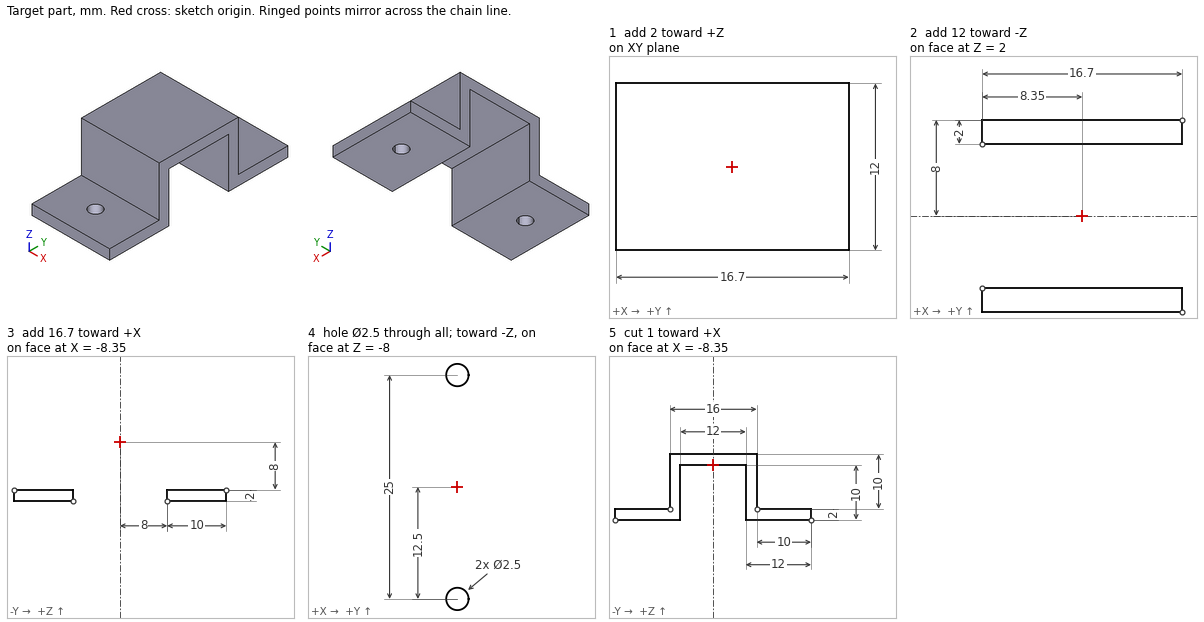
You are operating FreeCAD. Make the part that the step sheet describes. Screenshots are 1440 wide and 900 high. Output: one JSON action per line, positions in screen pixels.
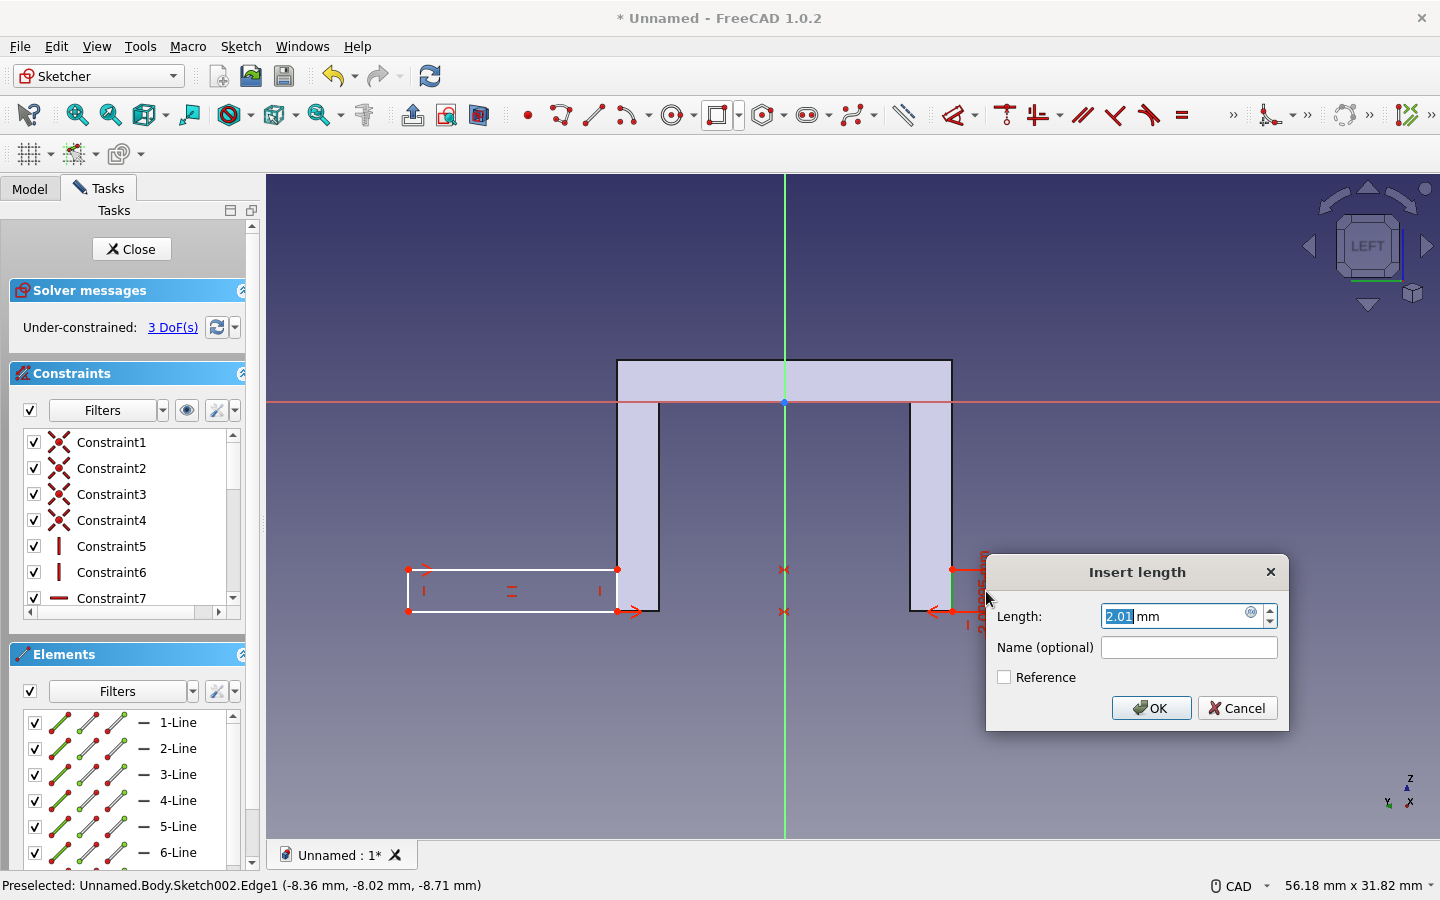
{"action": "type", "text": "2"}
{"action": "key", "text": "Return"}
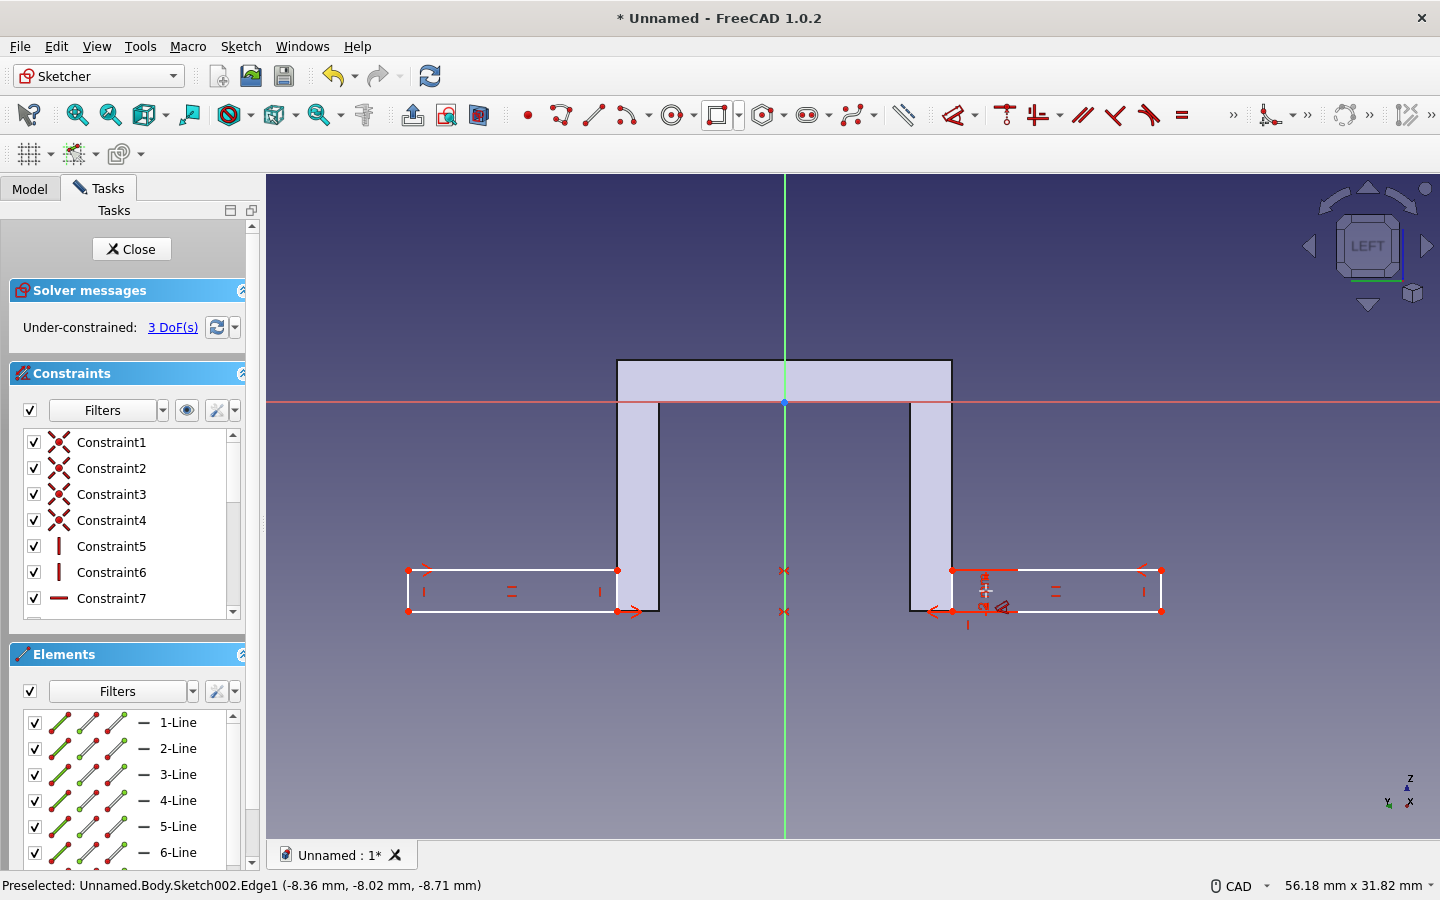
{"action": "left_click", "coordinate": [1015, 612]}
{"action": "left_click", "coordinate": [1057, 646]}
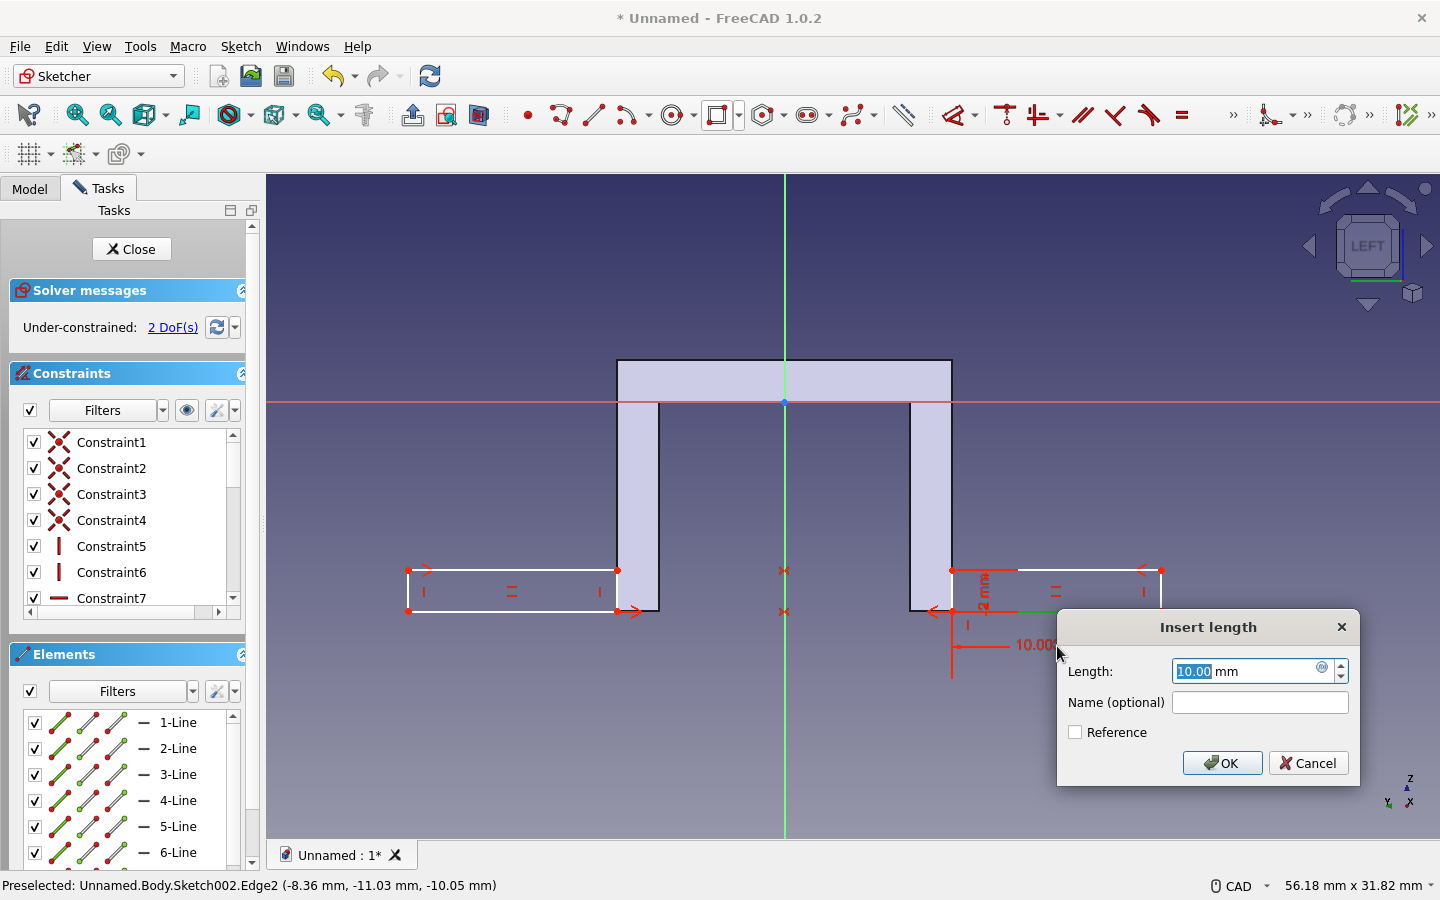
{"action": "type", "text": "10"}
{"action": "key", "text": "Return"}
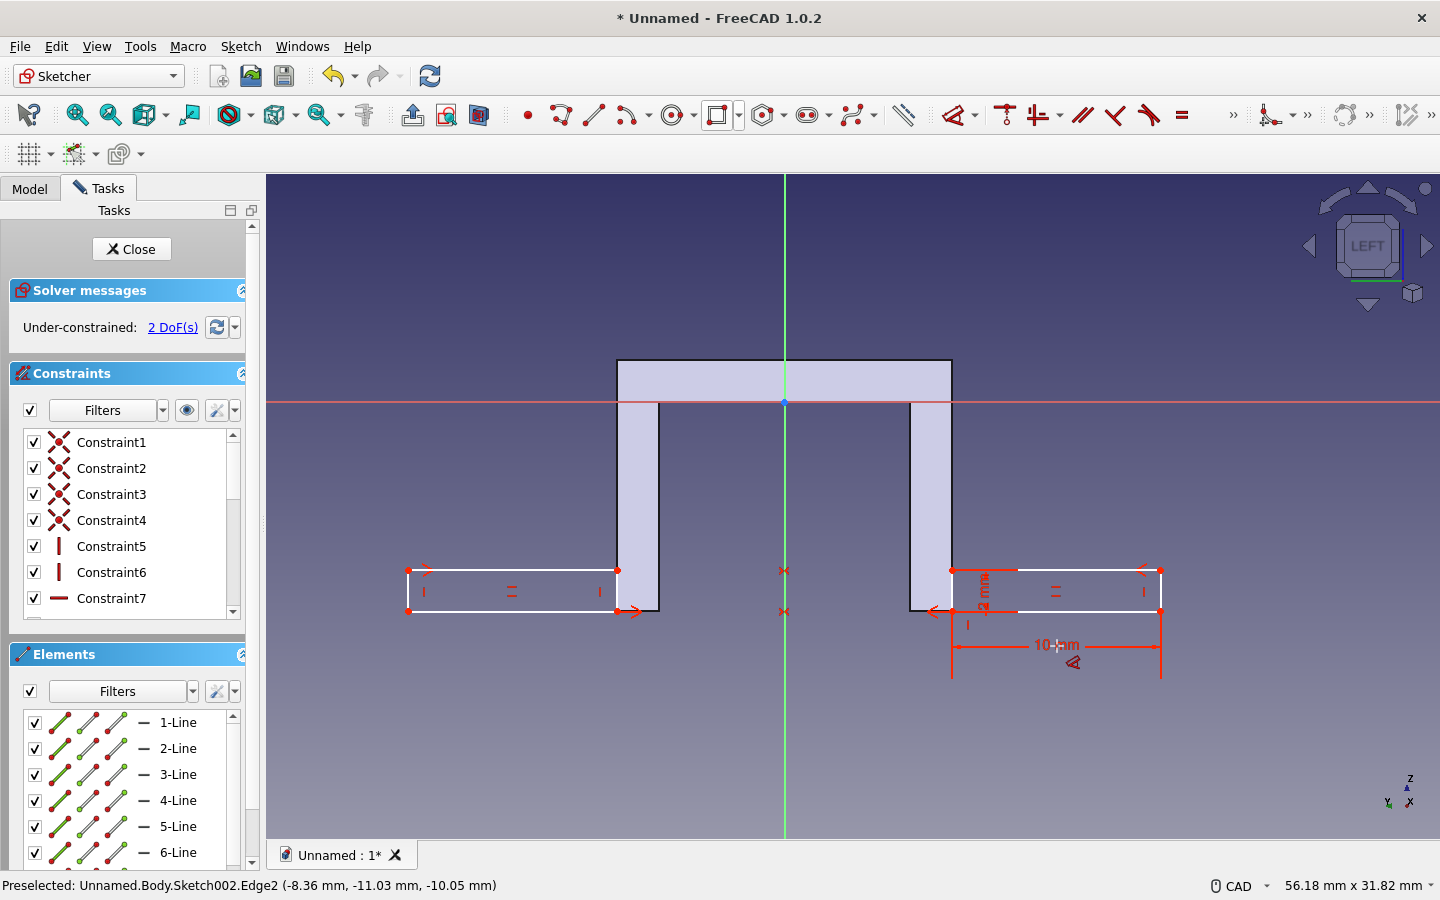
{"action": "left_click", "coordinate": [952, 570]}
{"action": "left_click", "coordinate": [868, 368]}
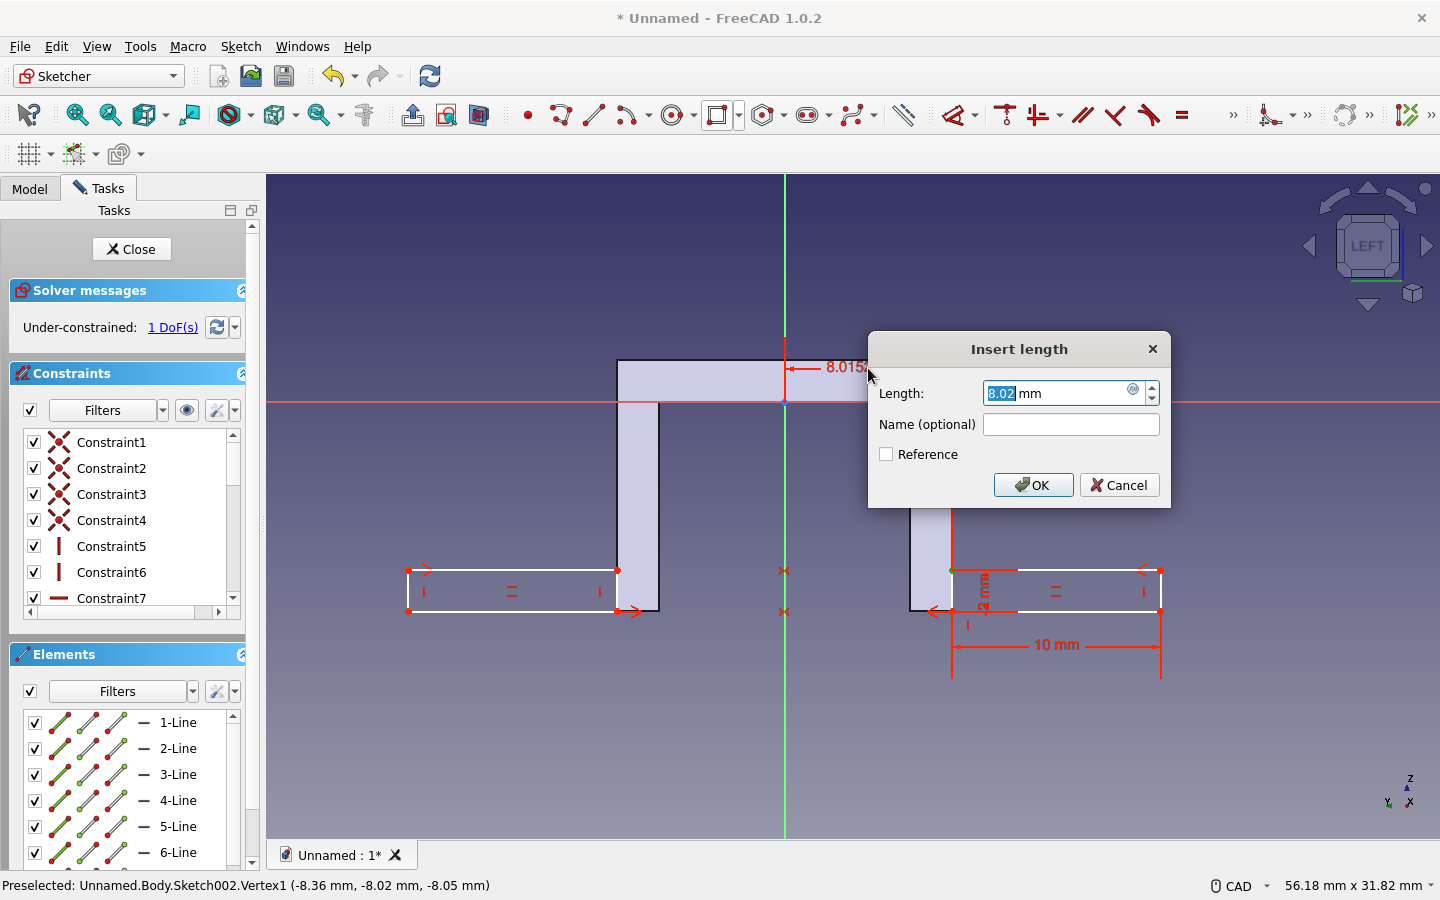
{"action": "type", "text": "8"}
{"action": "key", "text": "Return"}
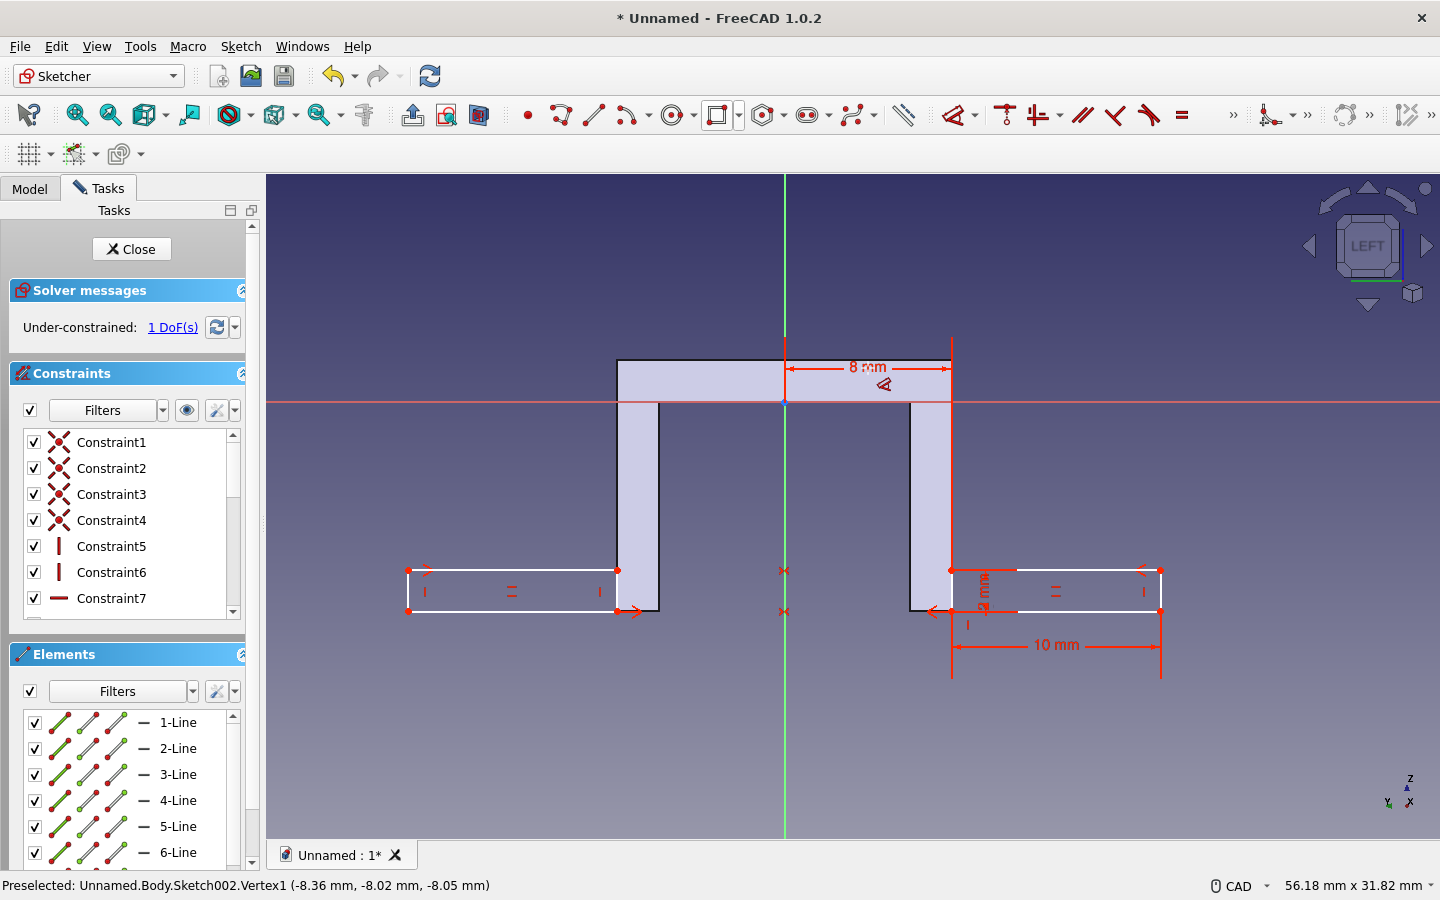
{"action": "left_click", "coordinate": [952, 570]}
{"action": "left_click", "coordinate": [986, 486]}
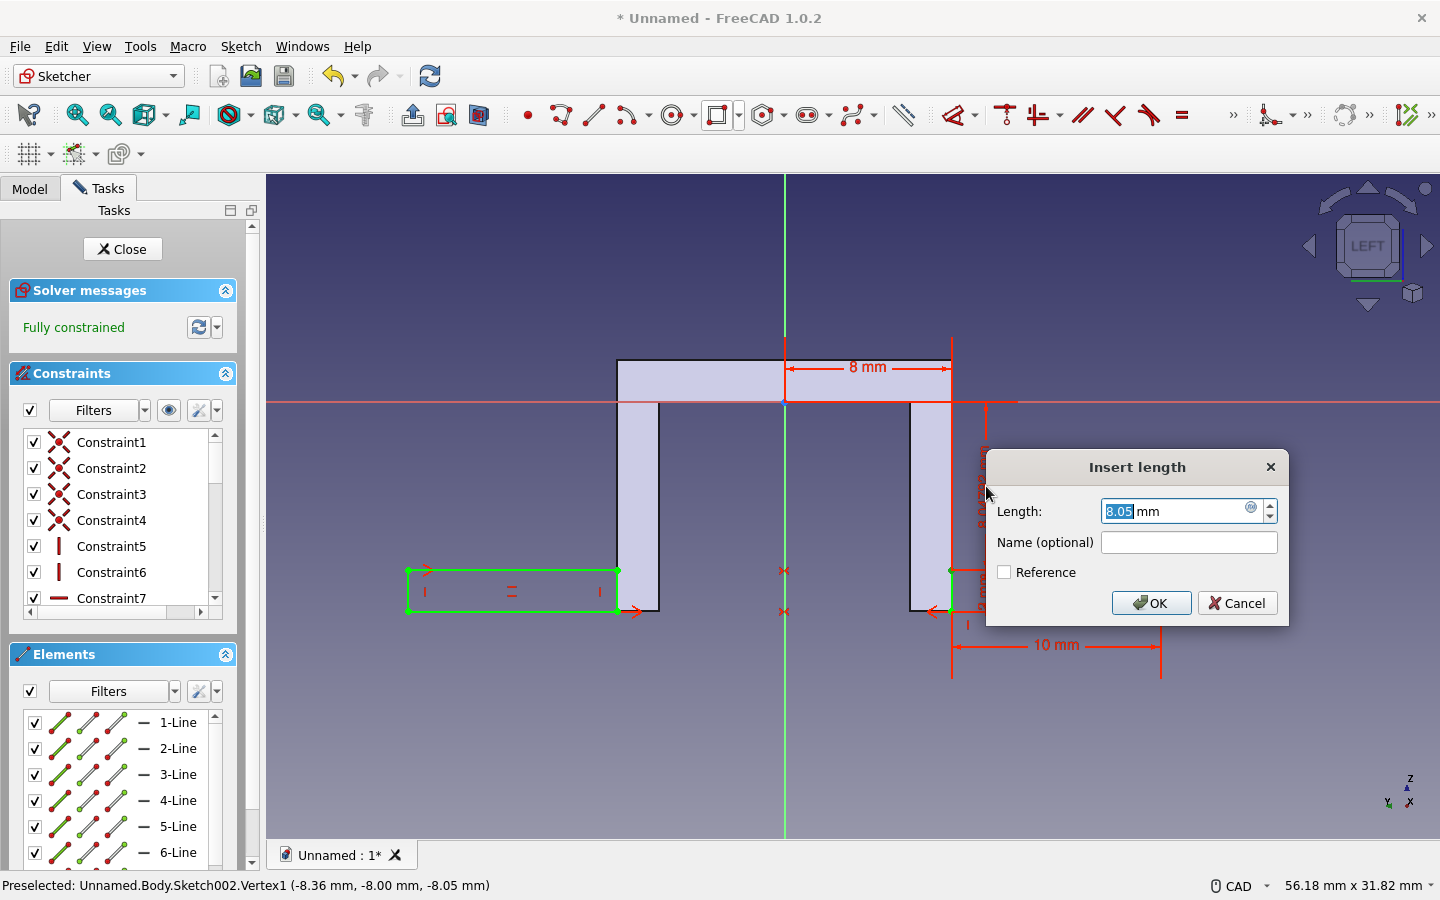
{"action": "type", "text": "8"}
{"action": "key", "text": "Return"}
{"action": "key", "text": "Escape"}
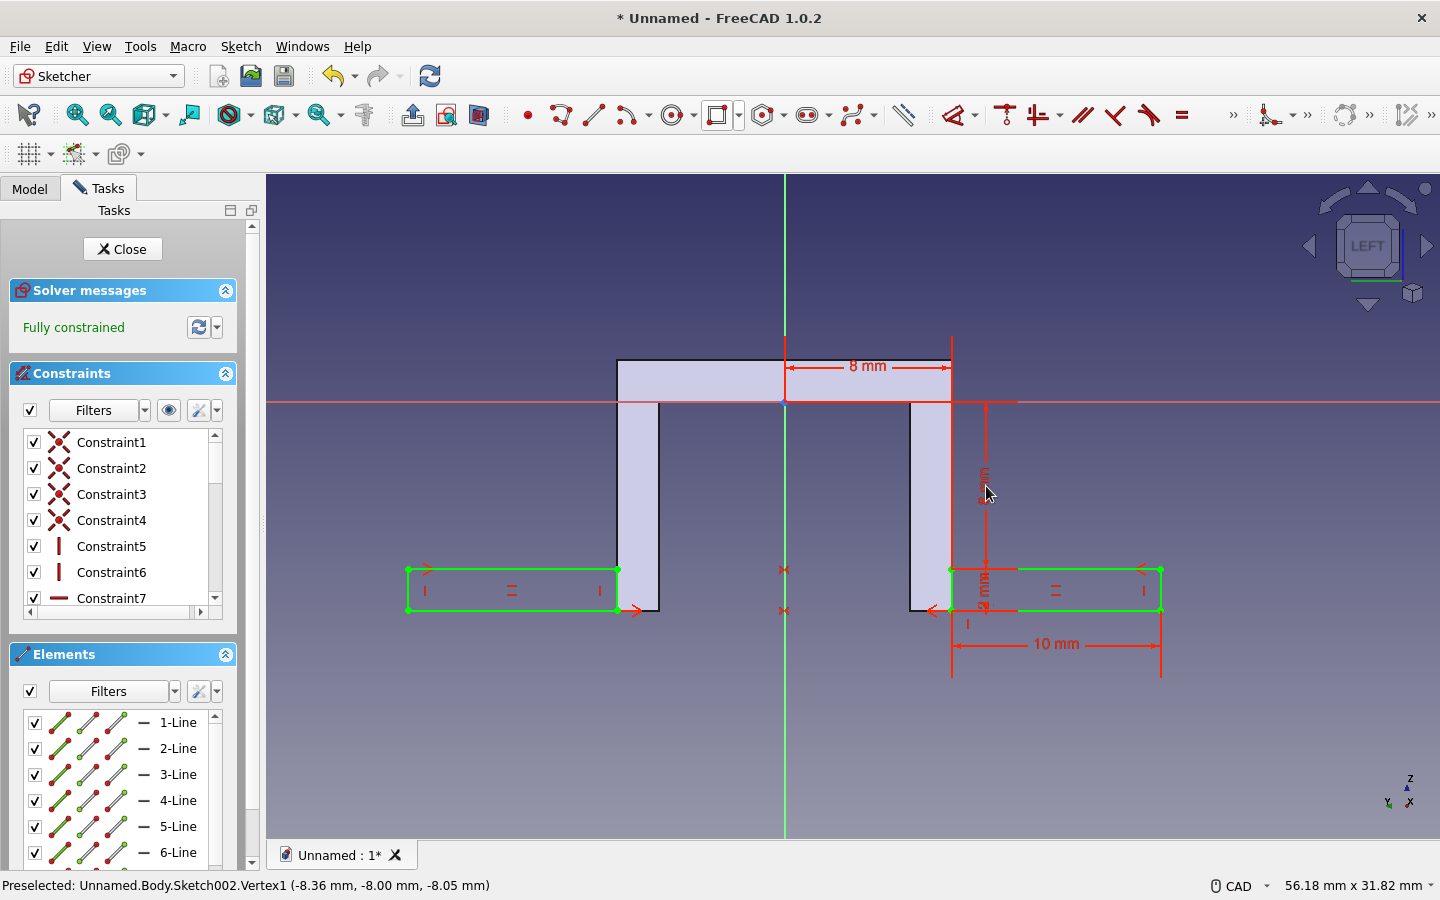
{"action": "left_click", "coordinate": [123, 249]}